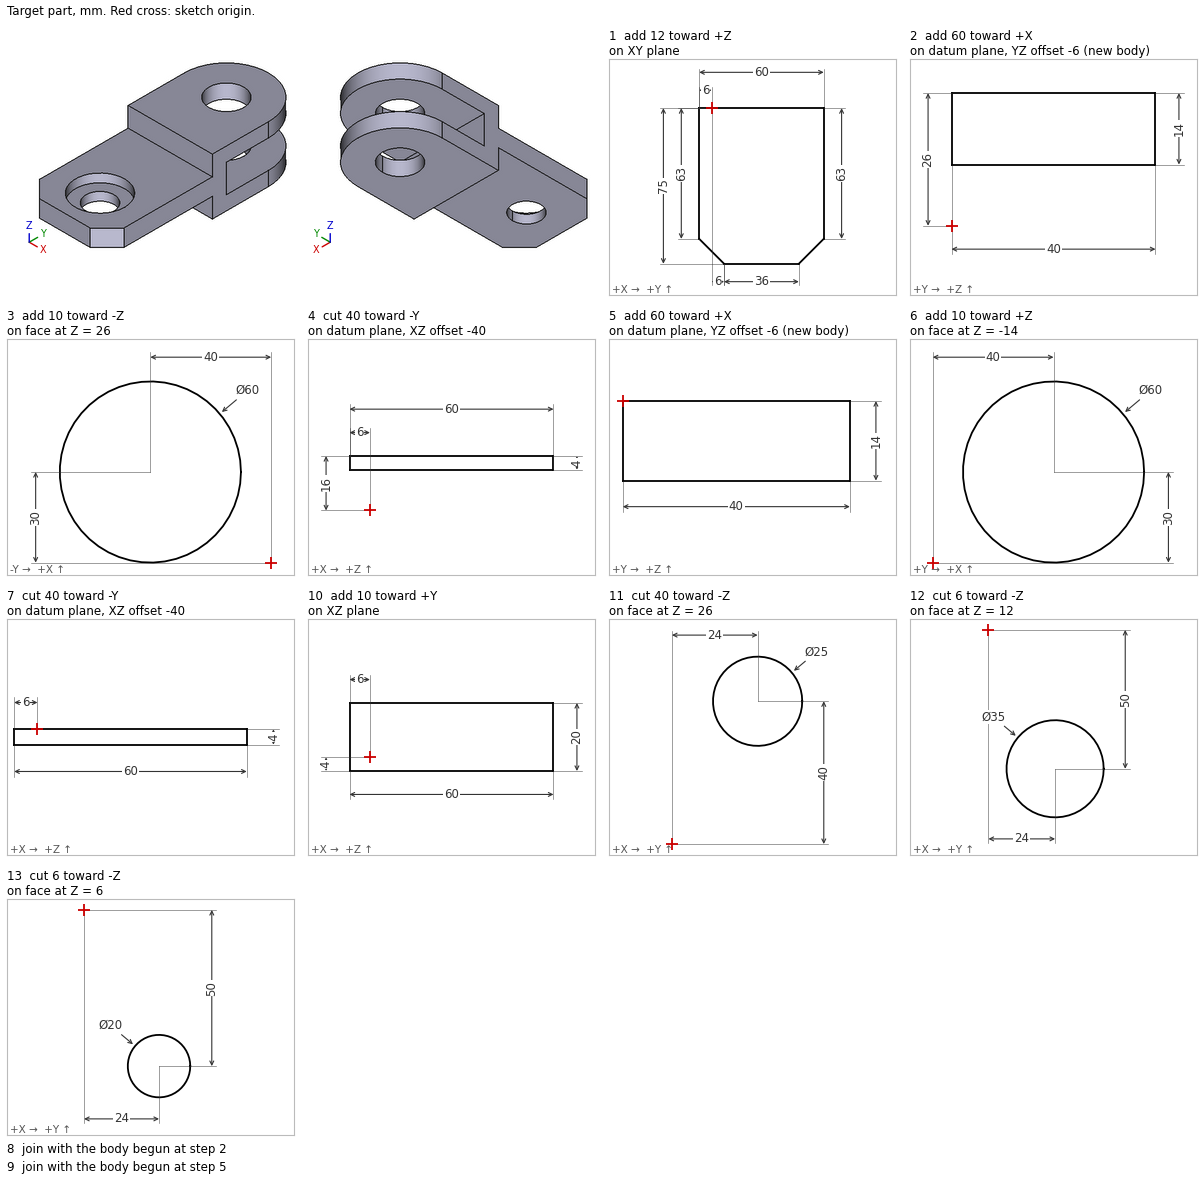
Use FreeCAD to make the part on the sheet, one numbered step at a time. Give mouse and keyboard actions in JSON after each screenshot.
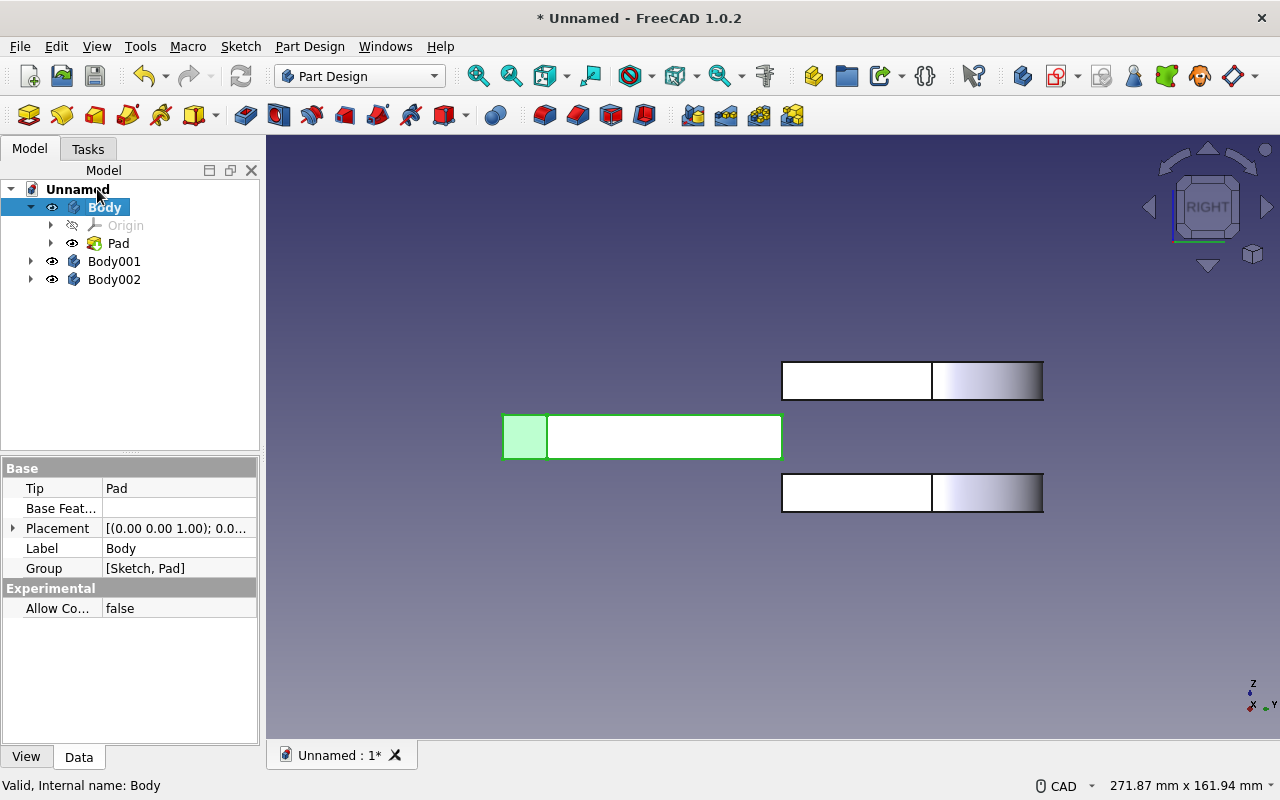
{"action": "left_click", "coordinate": [97, 207]}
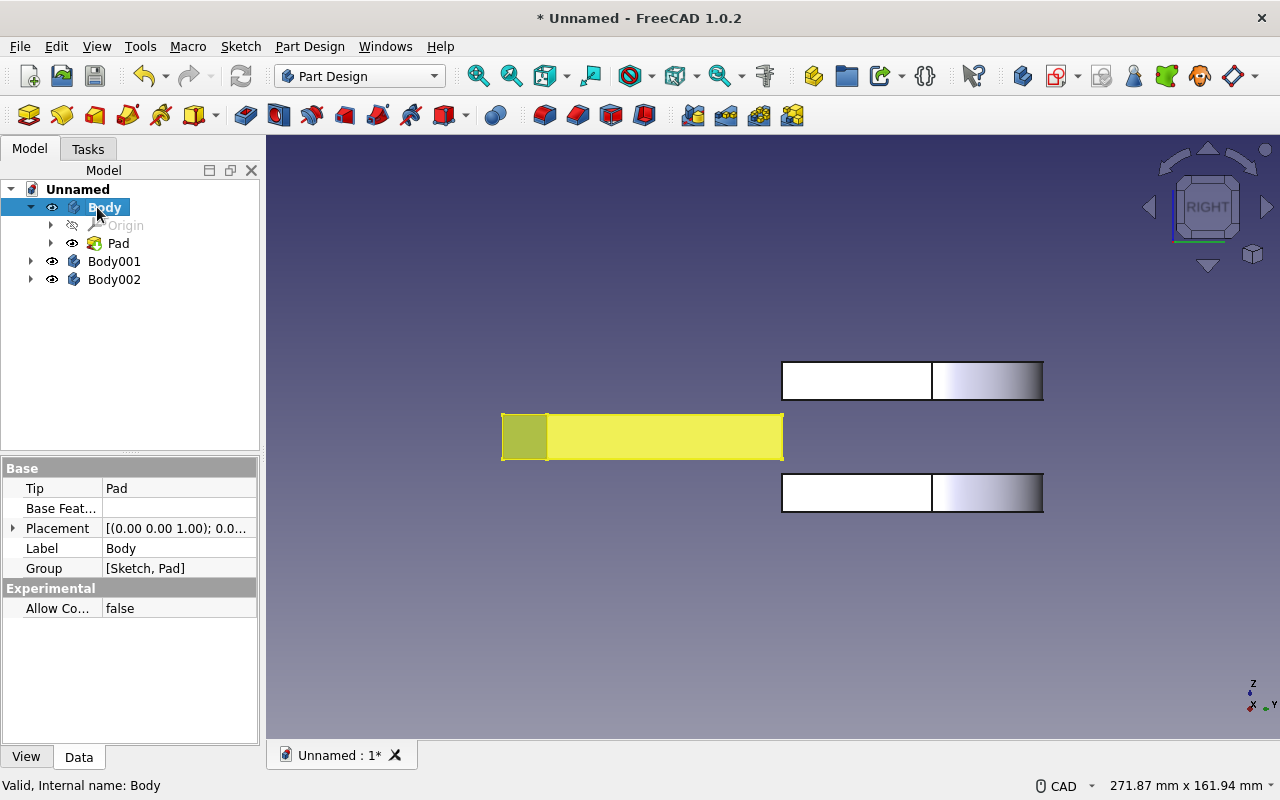
{"action": "left_click", "coordinate": [148, 608]}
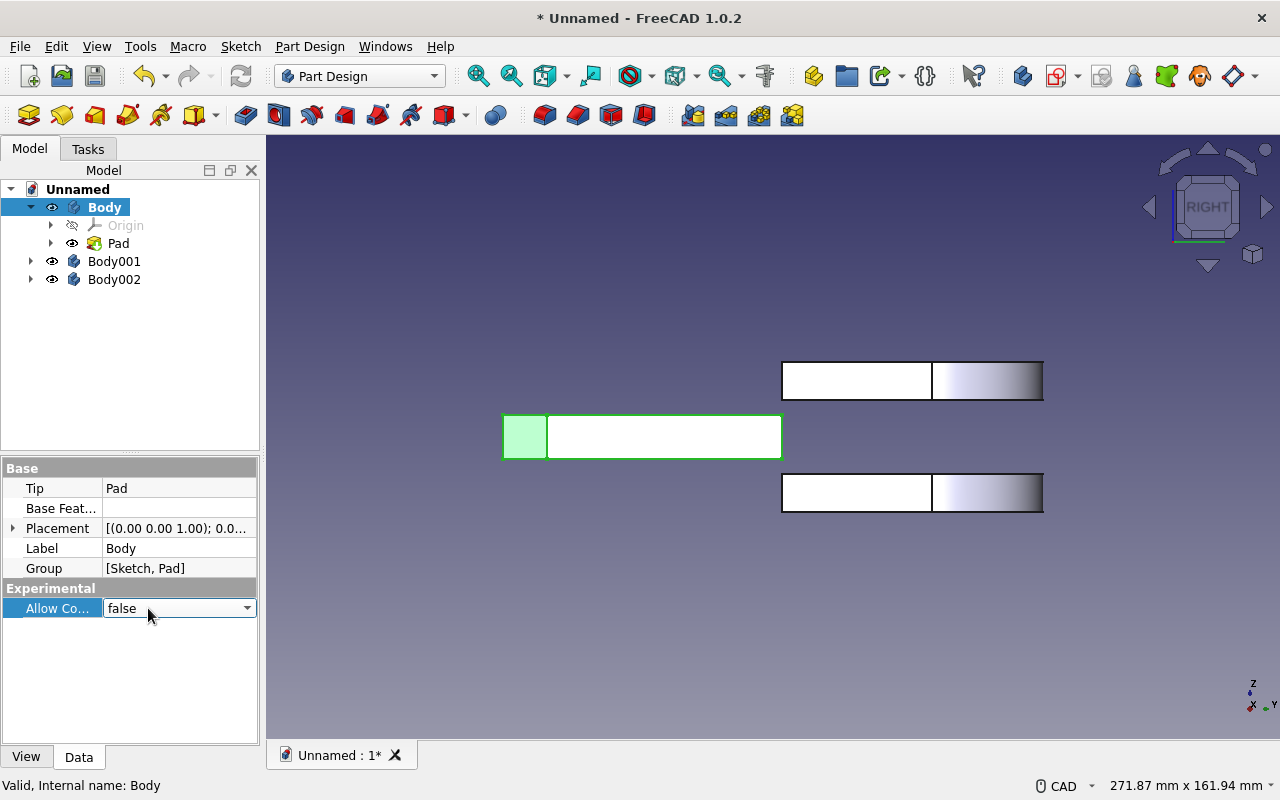
{"action": "left_click", "coordinate": [148, 608]}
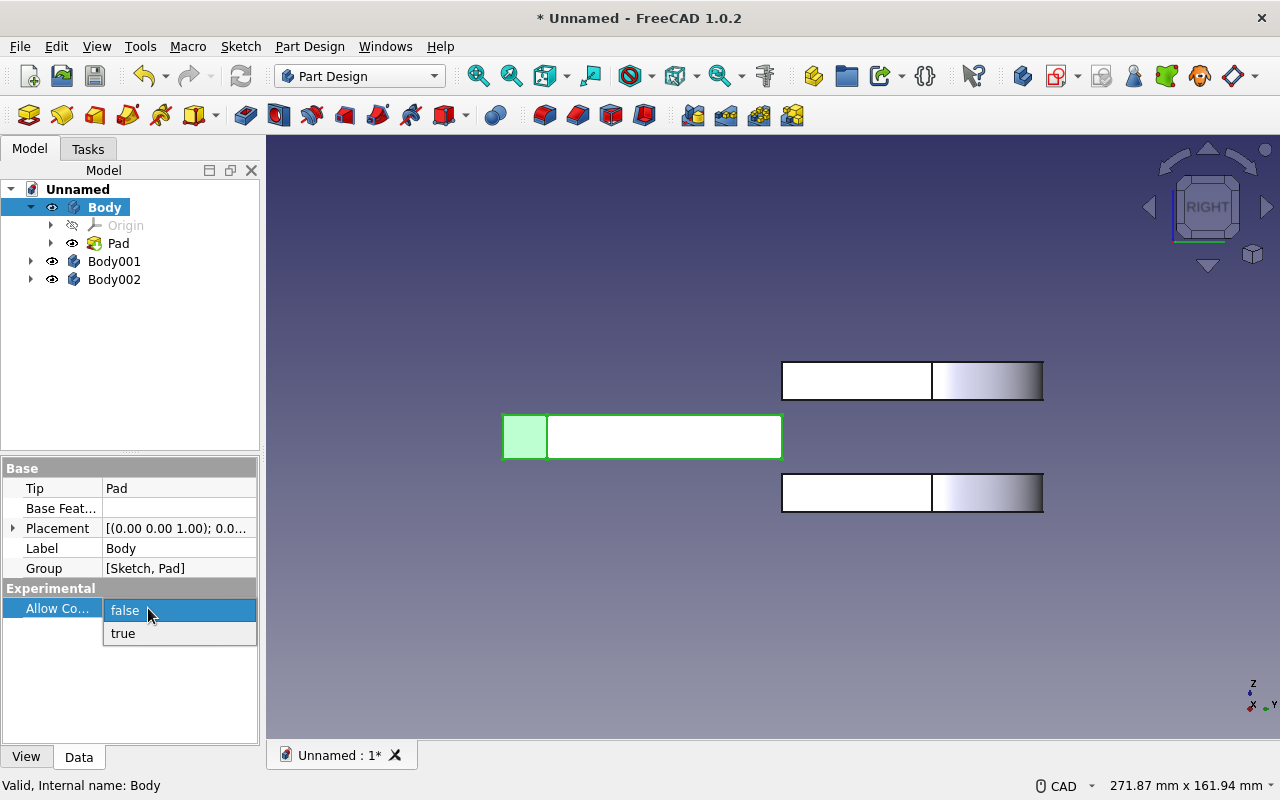
{"action": "left_click", "coordinate": [178, 634]}
{"action": "key", "text": "Return"}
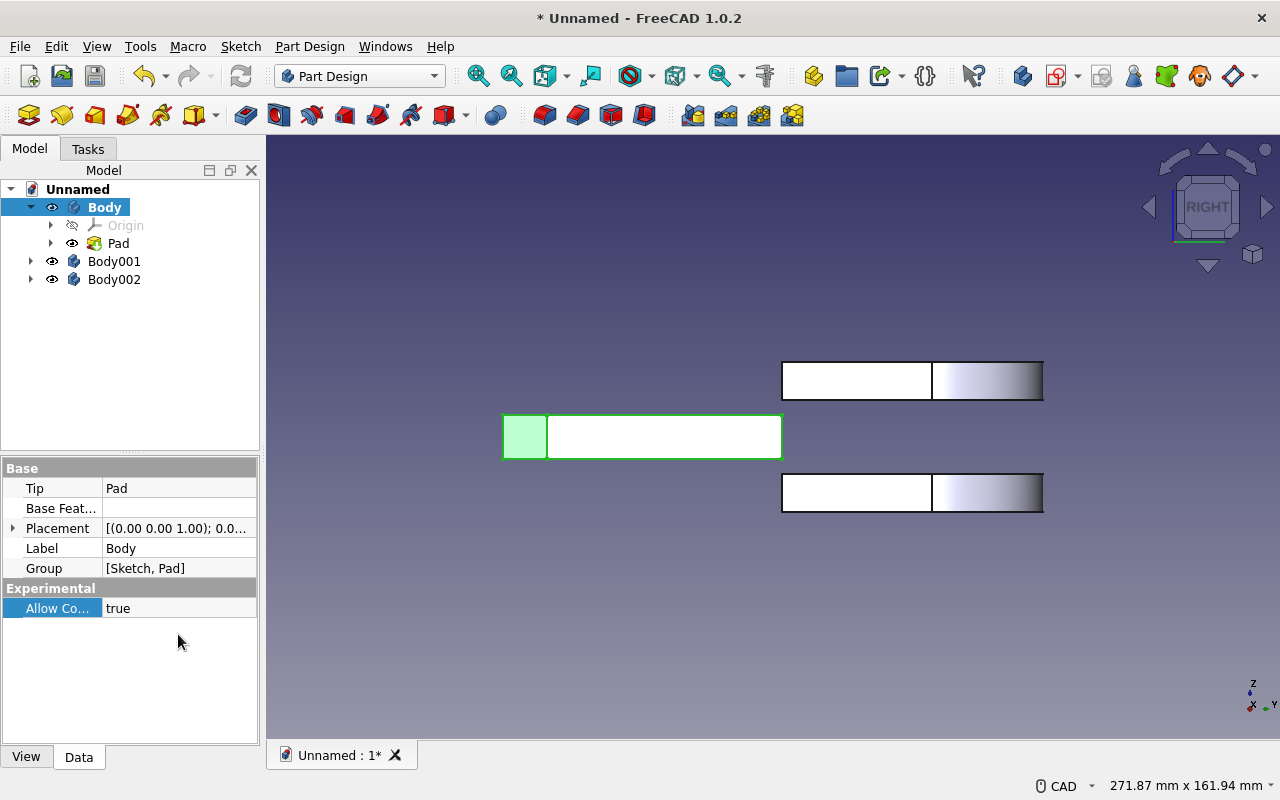
{"action": "left_click", "coordinate": [97, 261]}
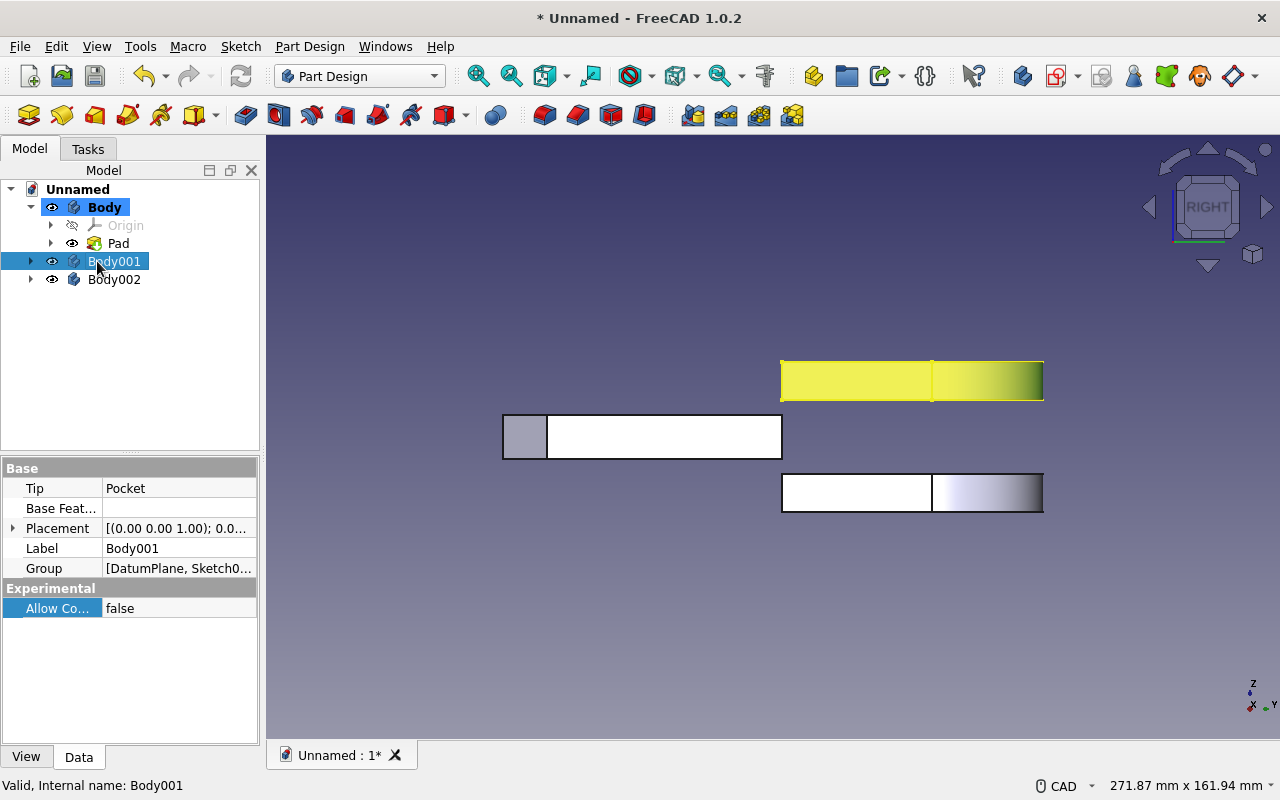
{"action": "left_click", "coordinate": [496, 116]}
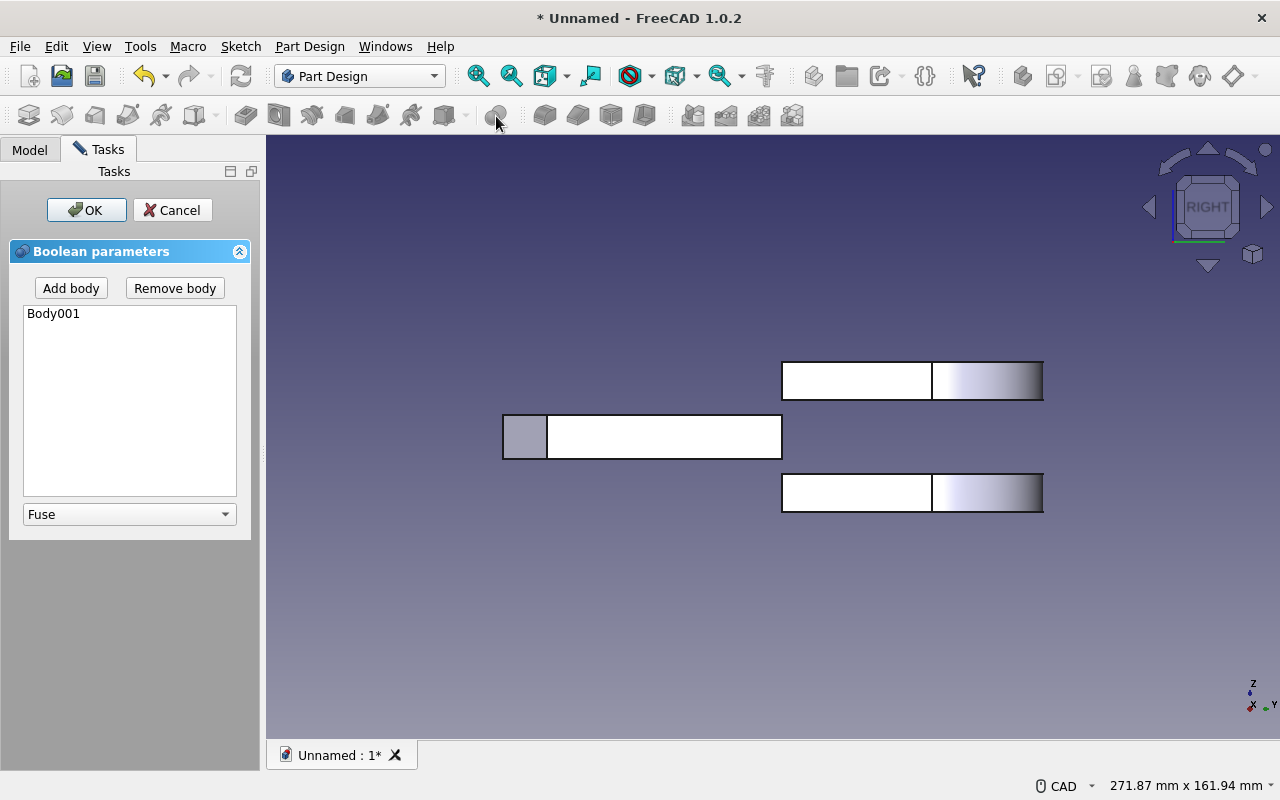
{"action": "left_click", "coordinate": [87, 210]}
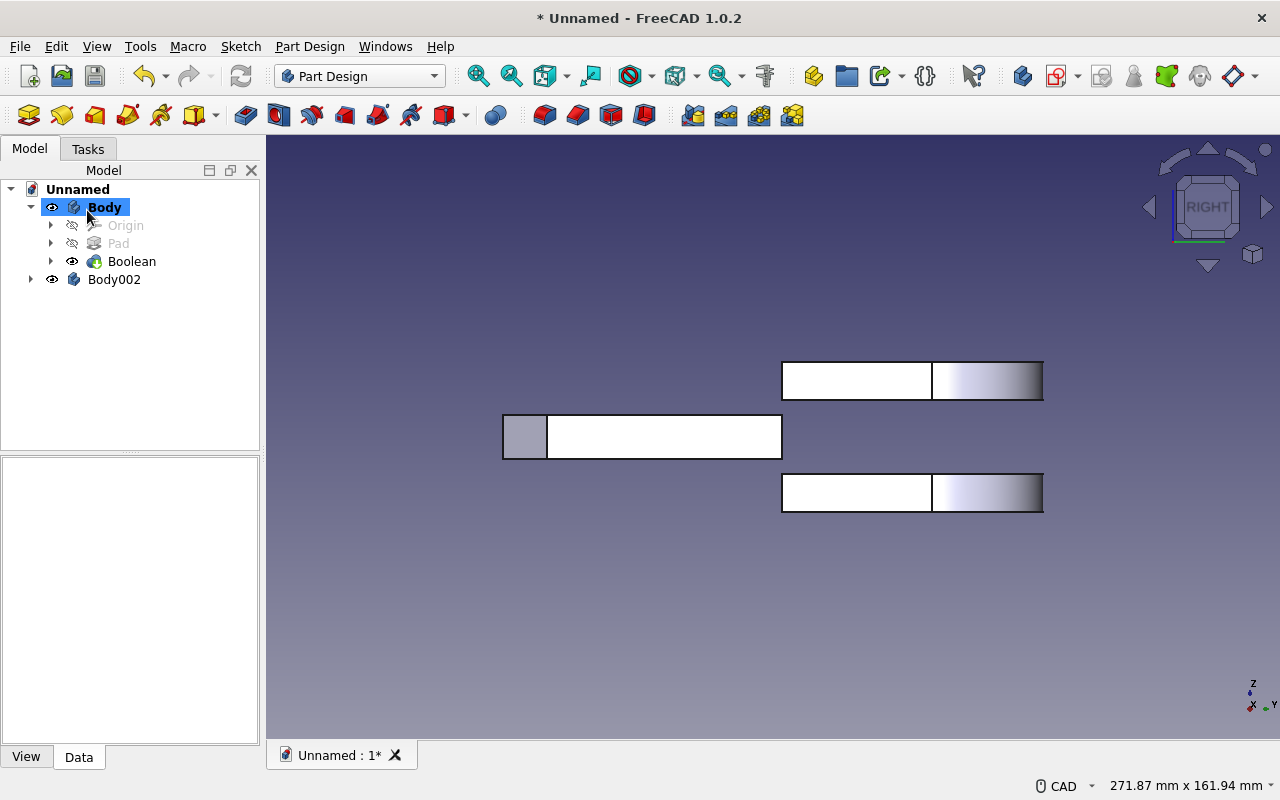
{"action": "left_click", "coordinate": [97, 279]}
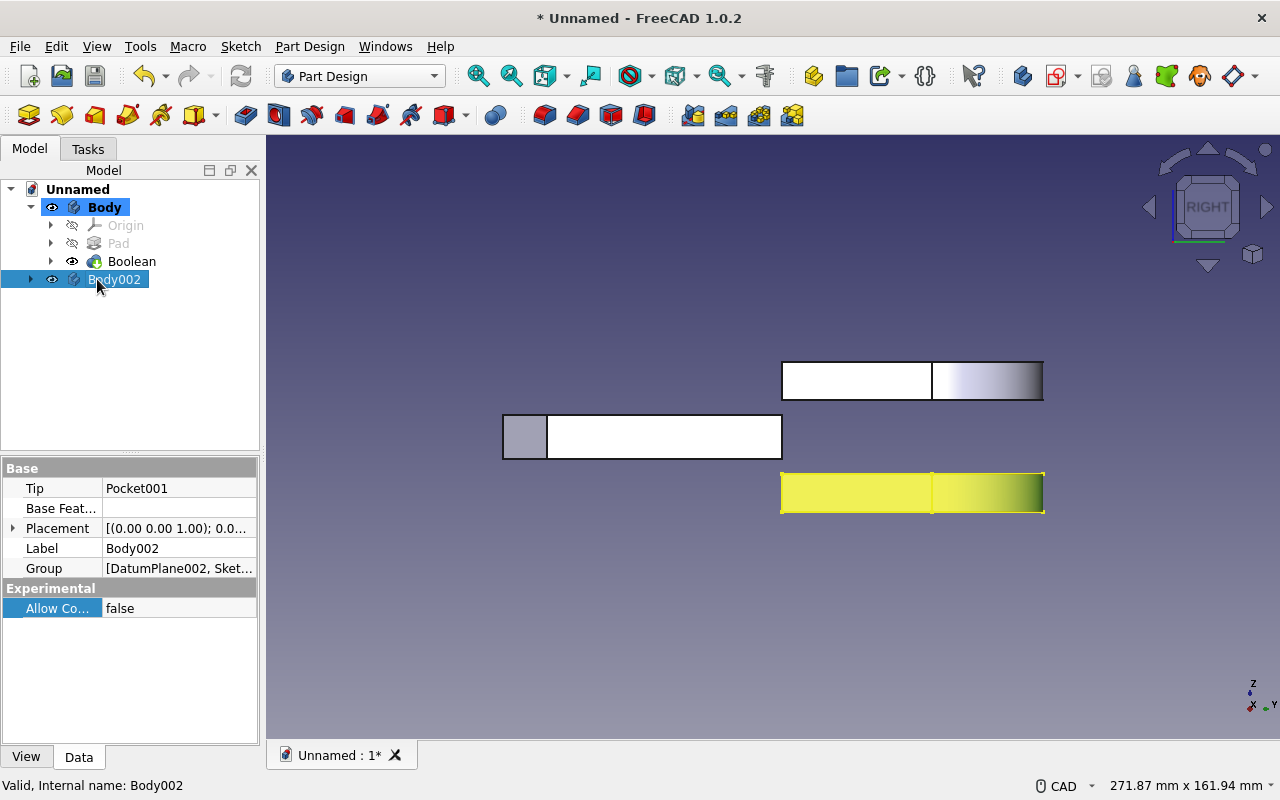
{"action": "left_click", "coordinate": [496, 116]}